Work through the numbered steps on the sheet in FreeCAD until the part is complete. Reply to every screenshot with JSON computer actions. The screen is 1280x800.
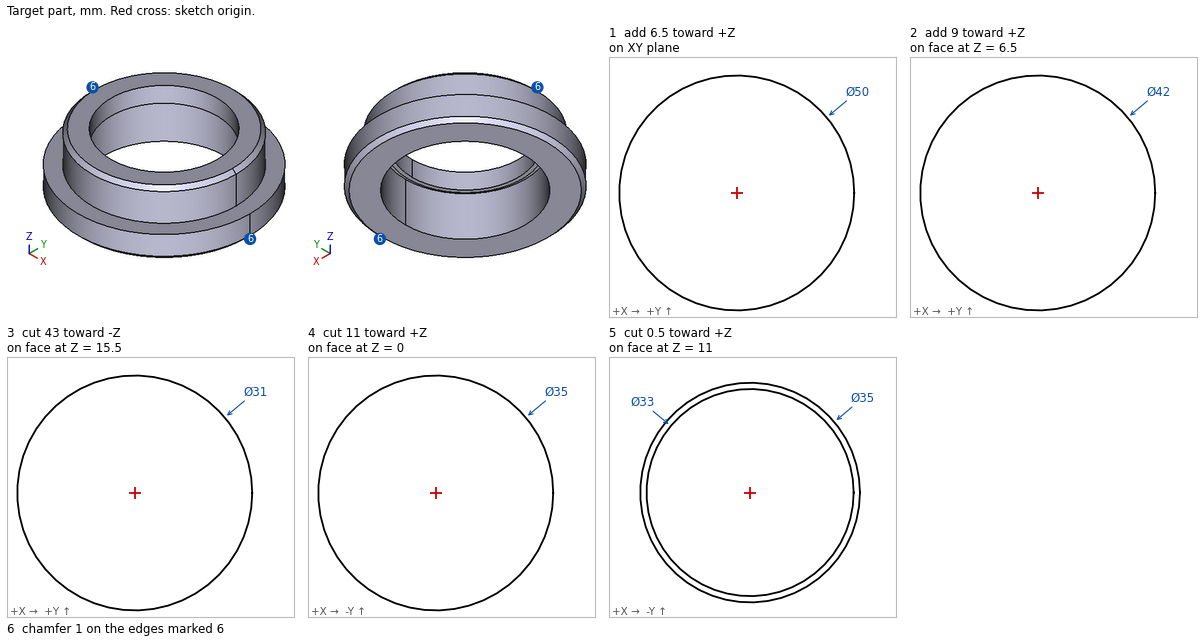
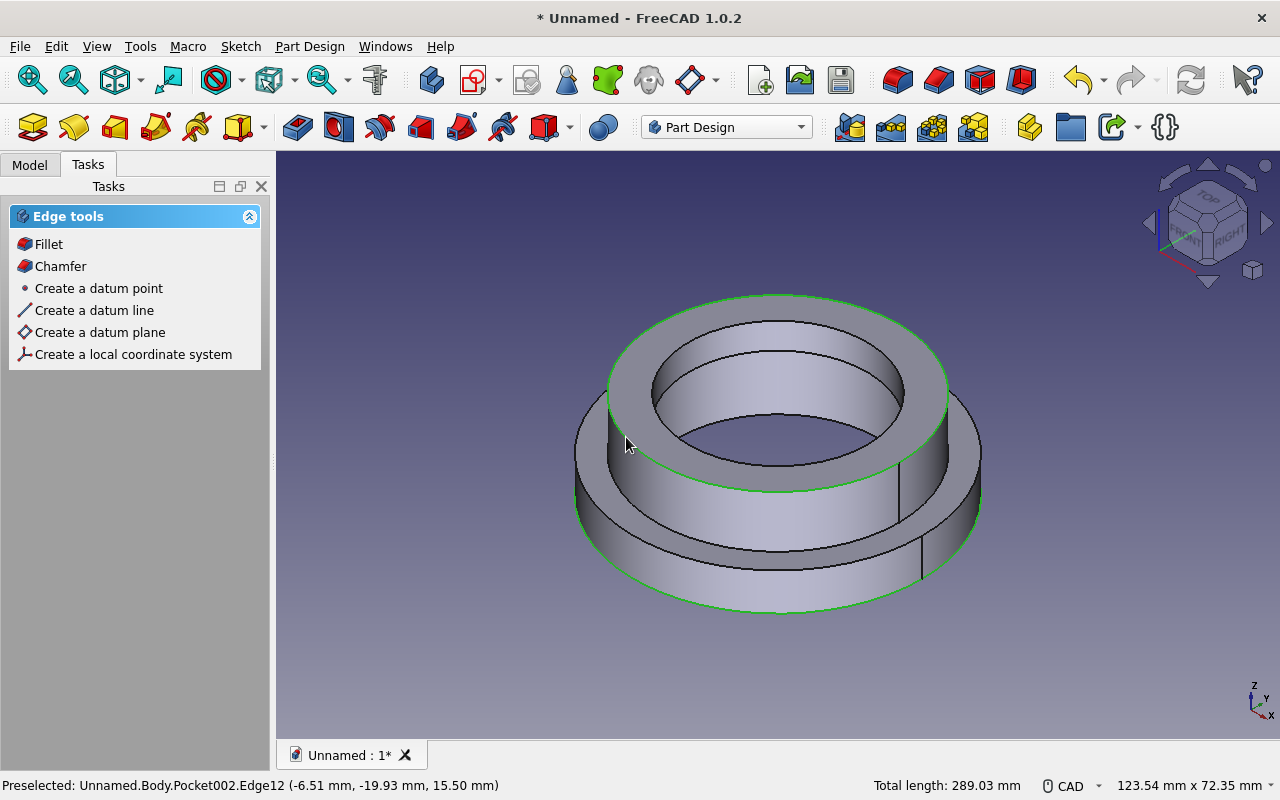
{"action": "left_click", "coordinate": [939, 80]}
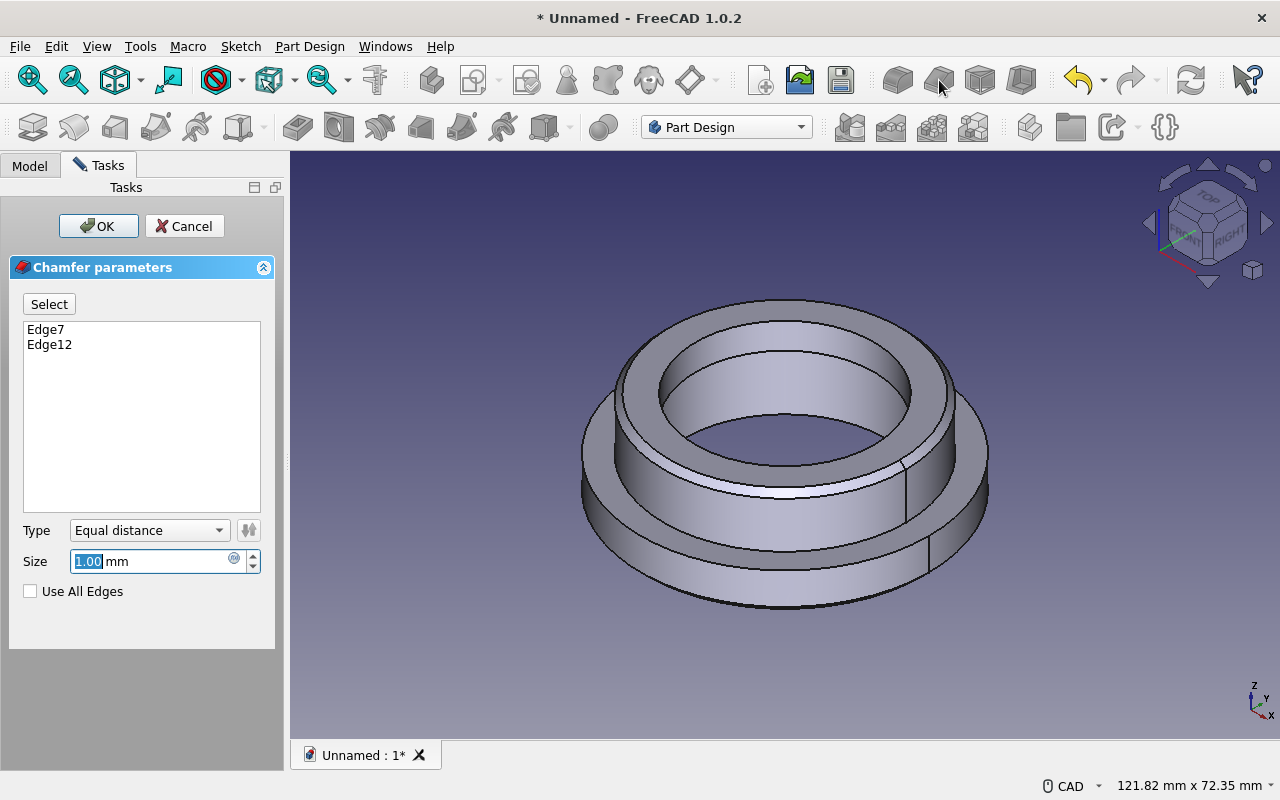
{"action": "type", "text": "1"}
{"action": "key", "text": "Tab"}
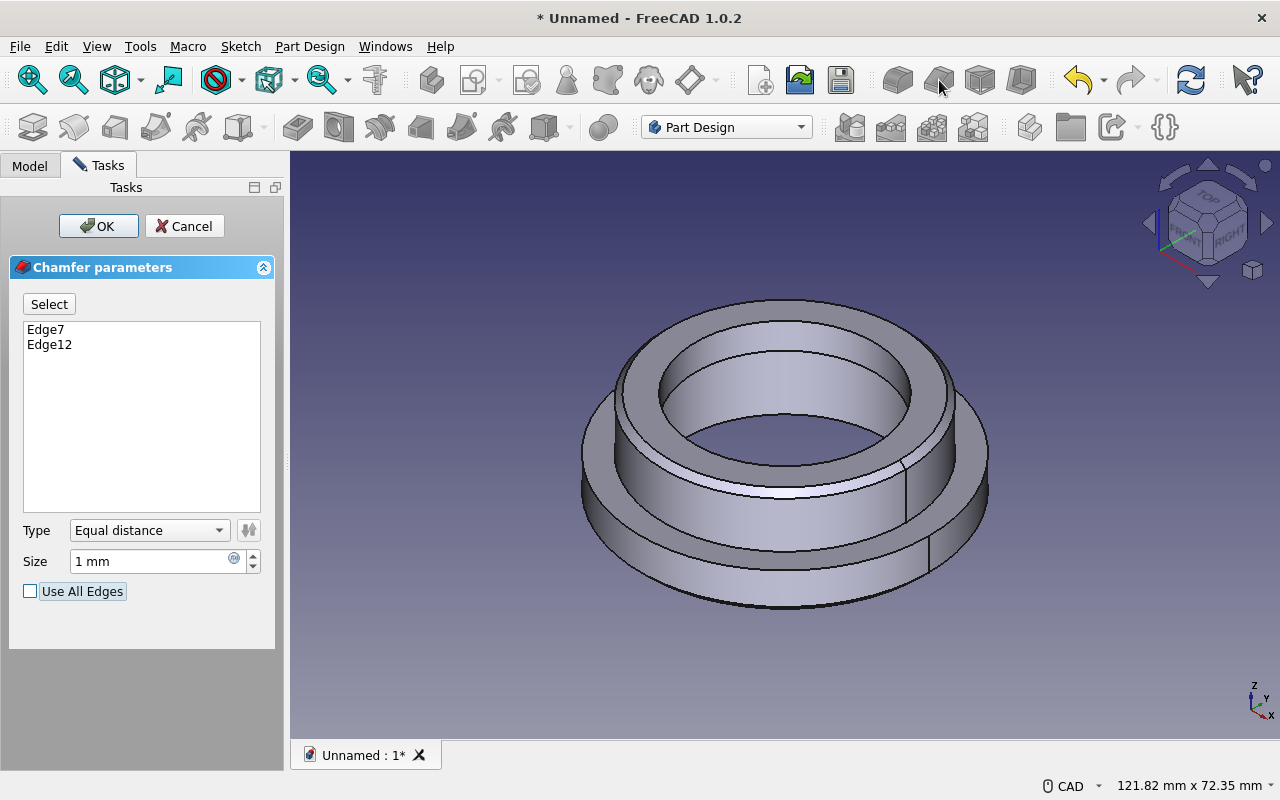
{"action": "left_click", "coordinate": [99, 226]}